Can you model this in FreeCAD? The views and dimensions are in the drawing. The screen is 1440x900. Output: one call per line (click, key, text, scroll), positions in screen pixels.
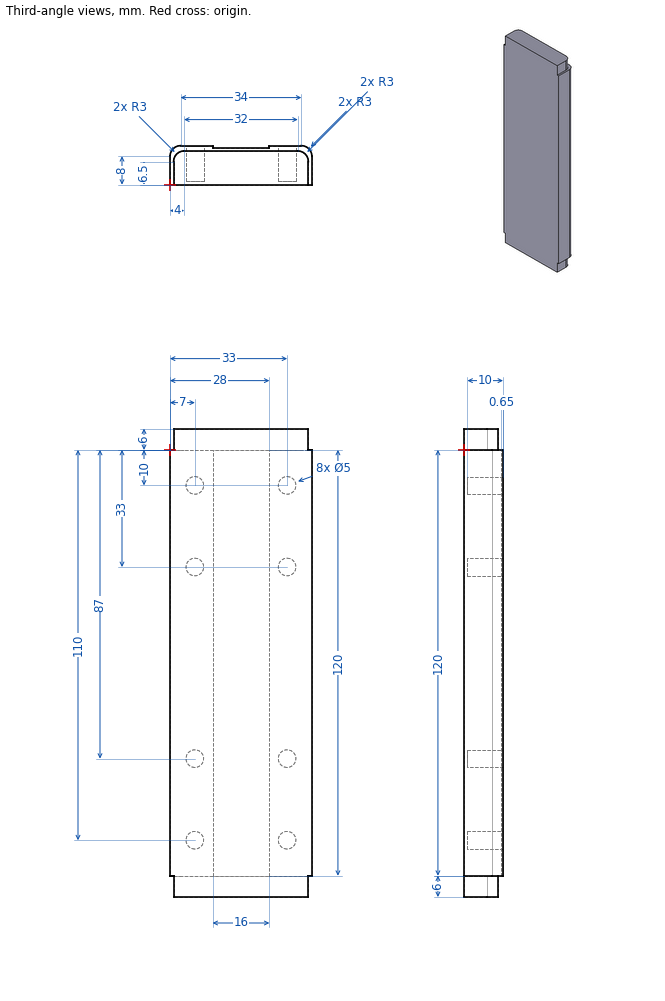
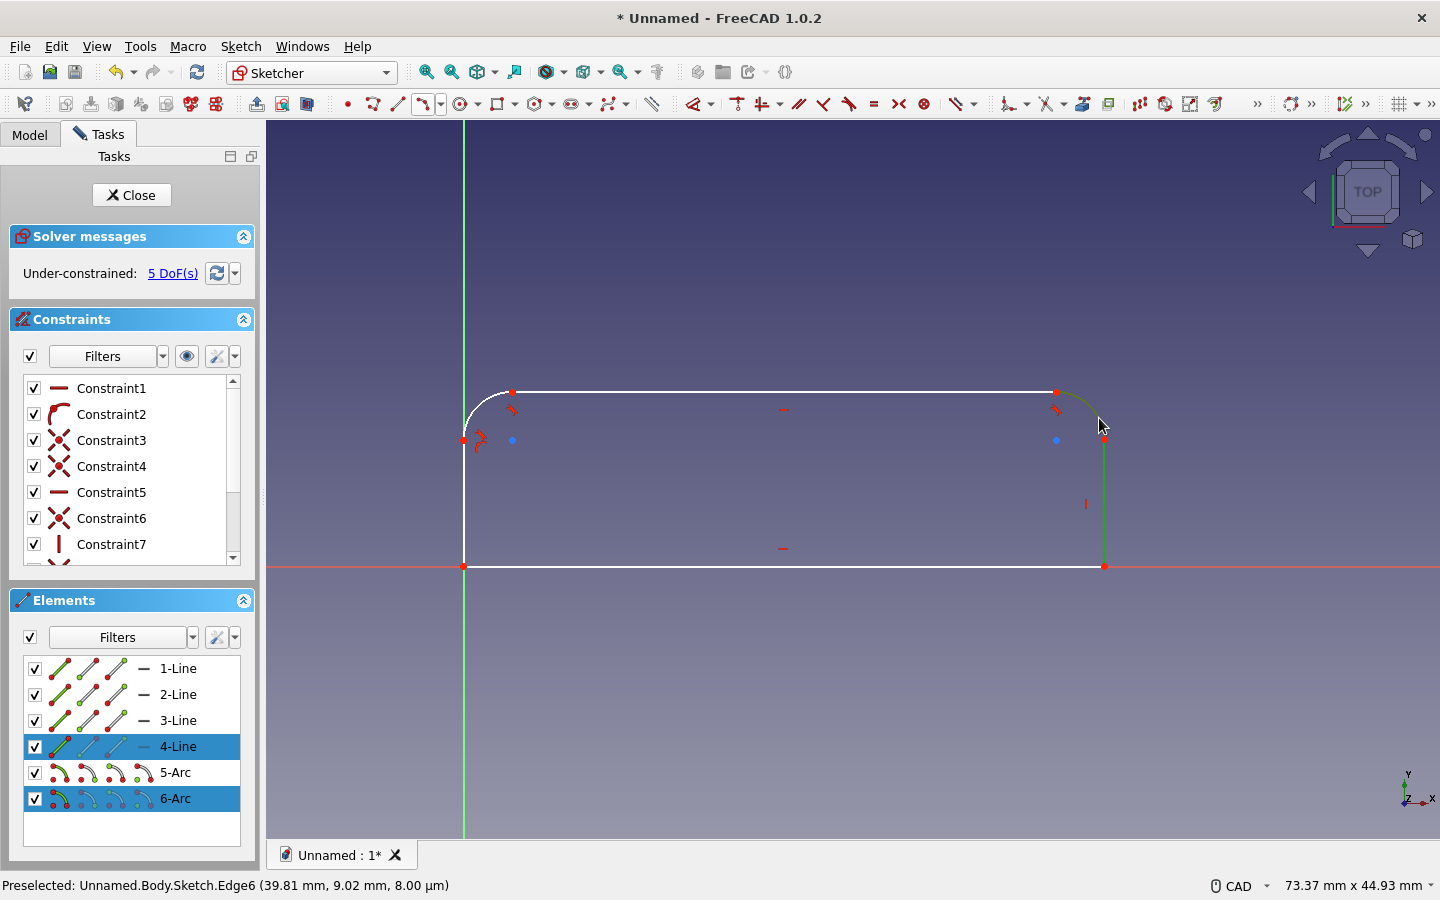
click(849, 104)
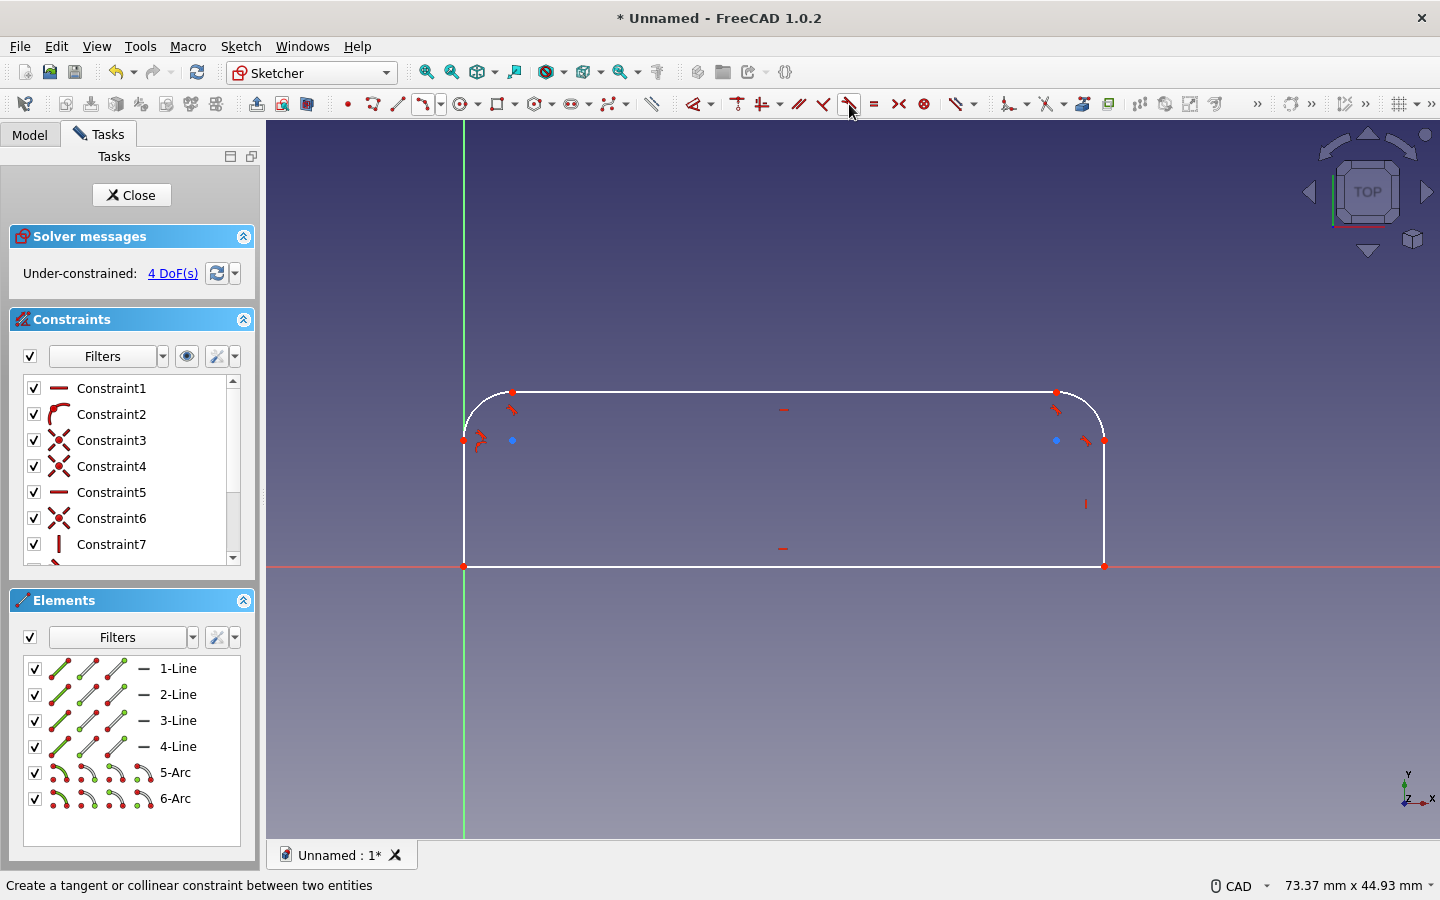
click(490, 397)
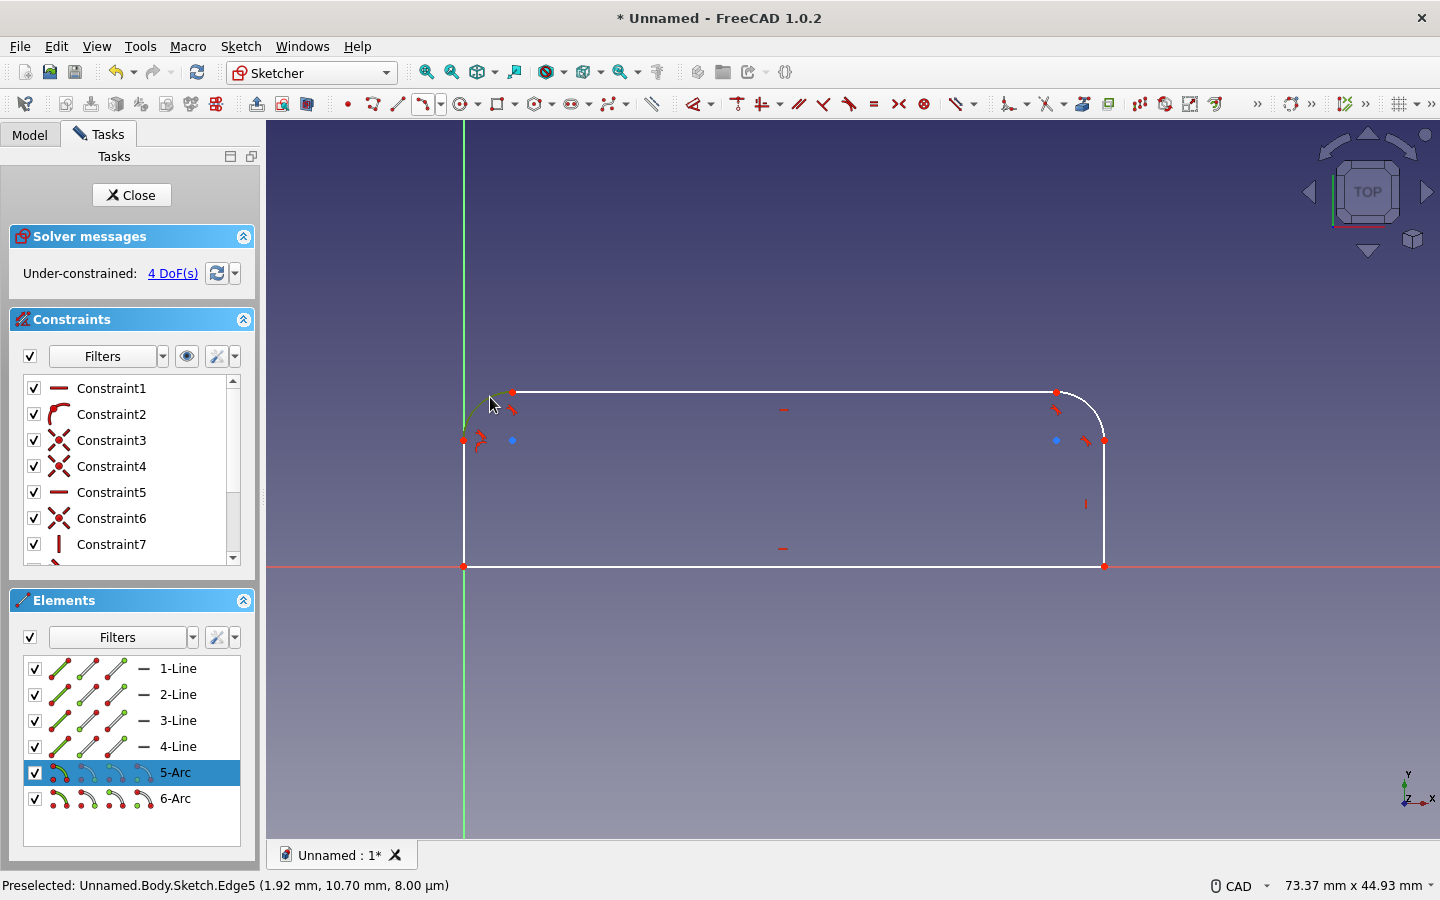
click(1099, 418)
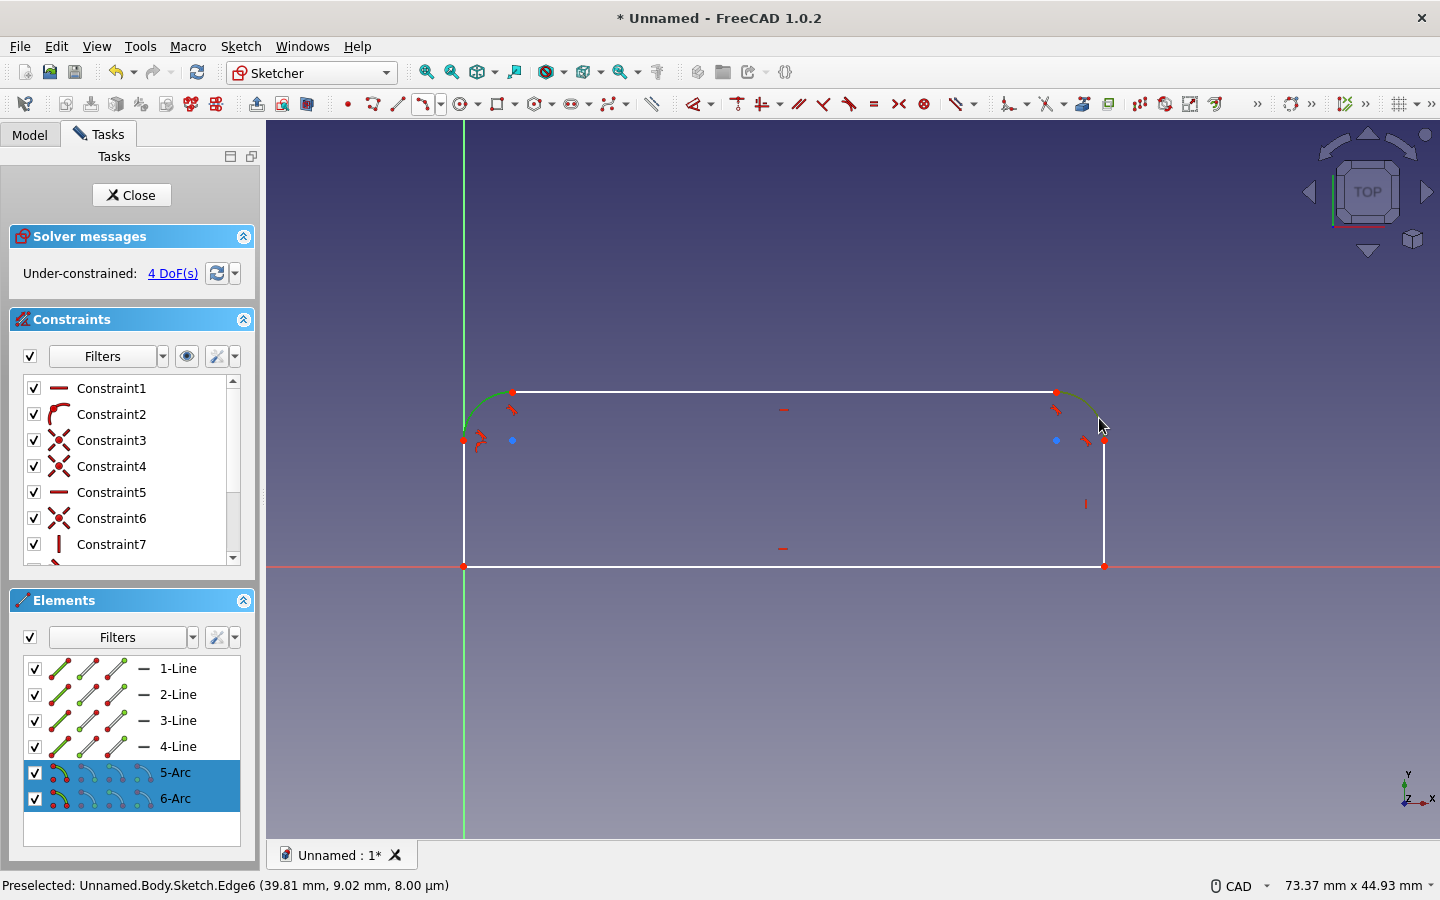
click(874, 104)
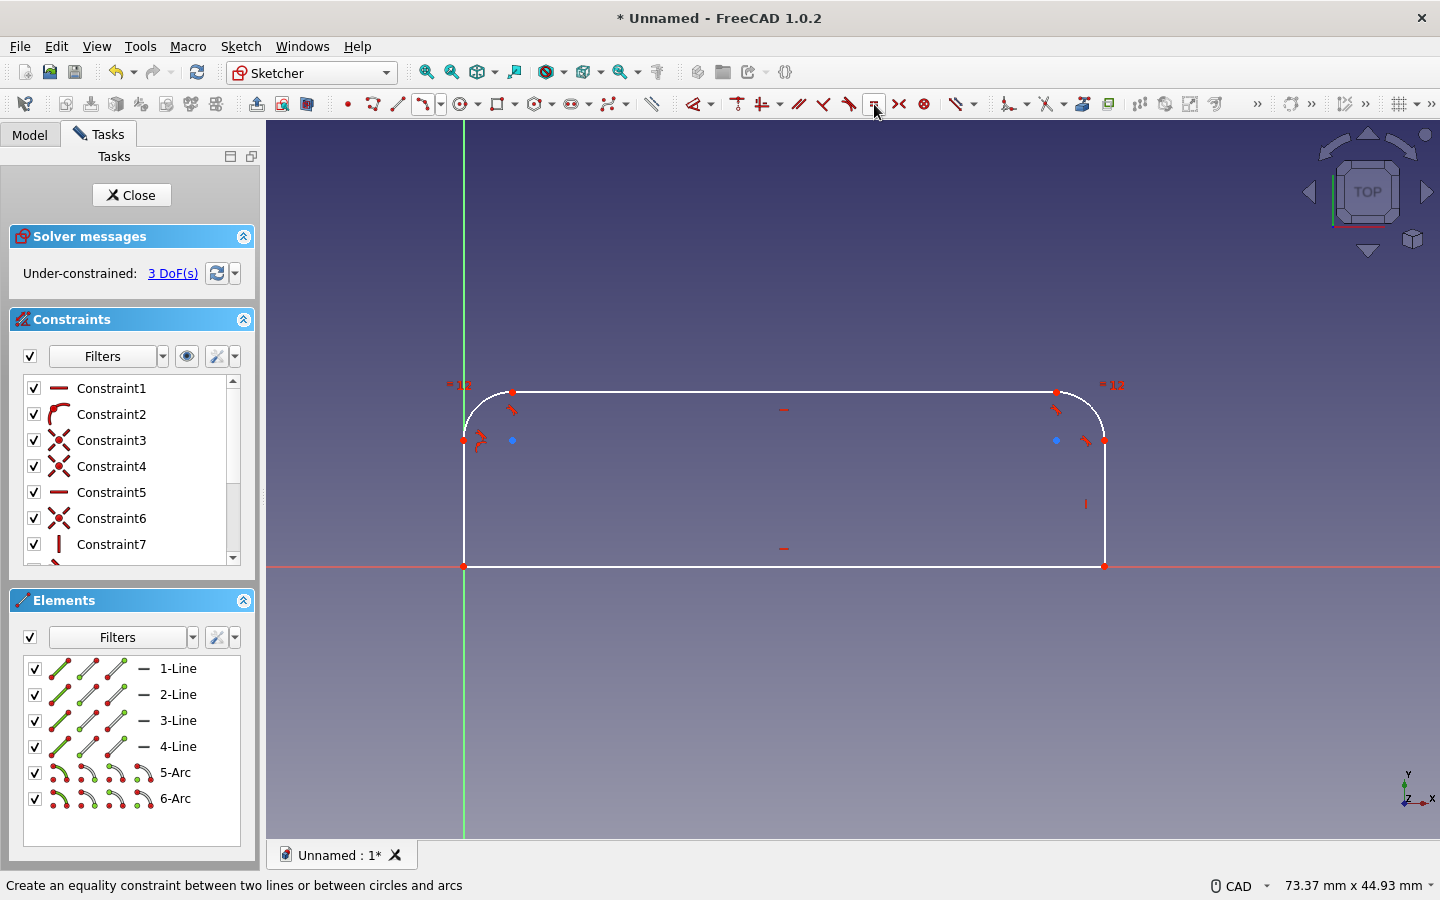
click(692, 104)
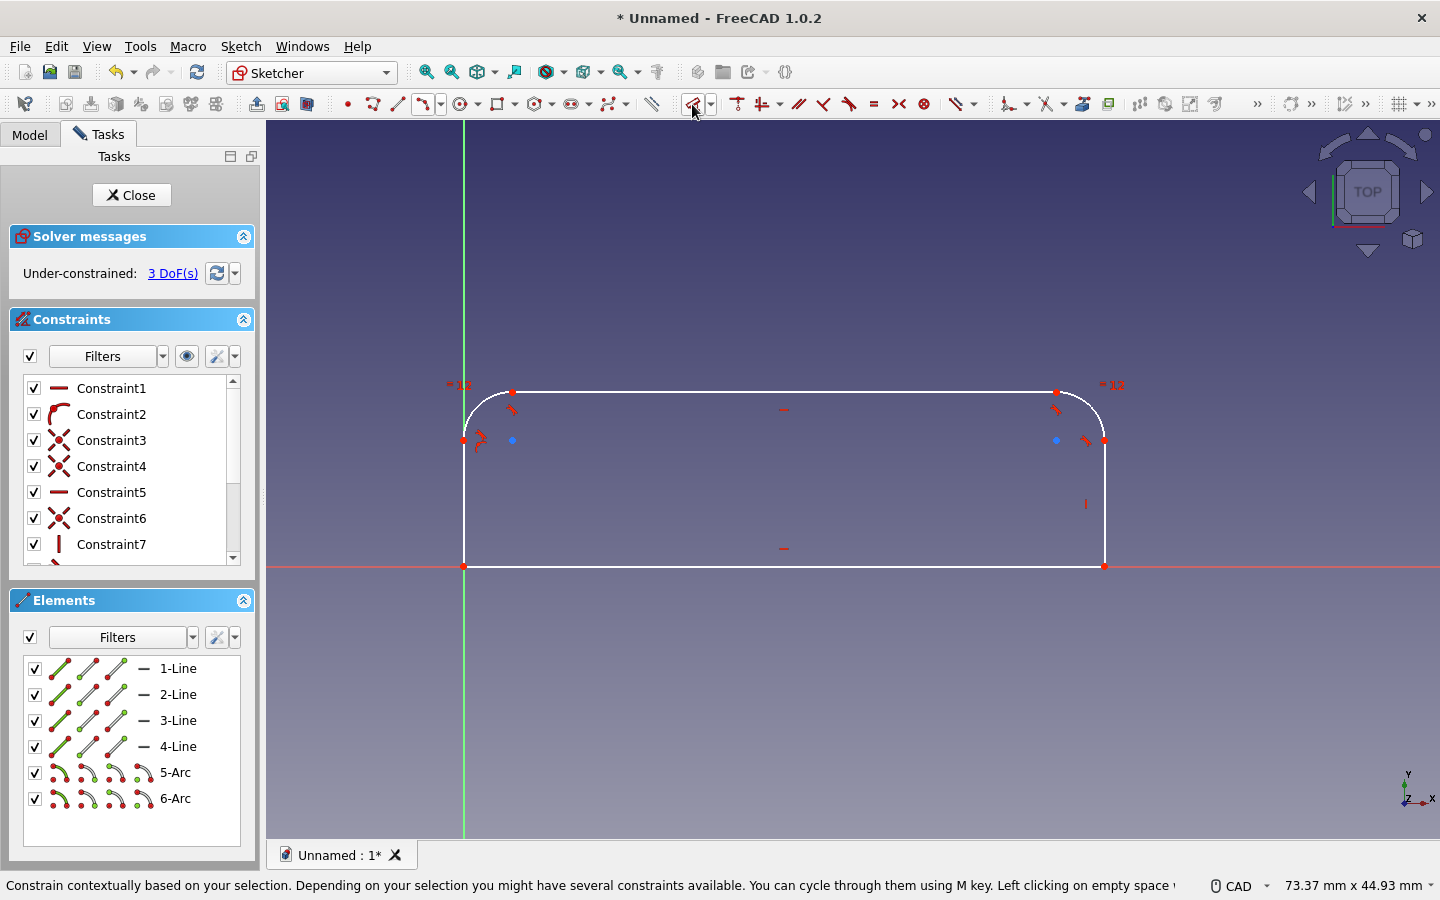
click(490, 397)
click(515, 360)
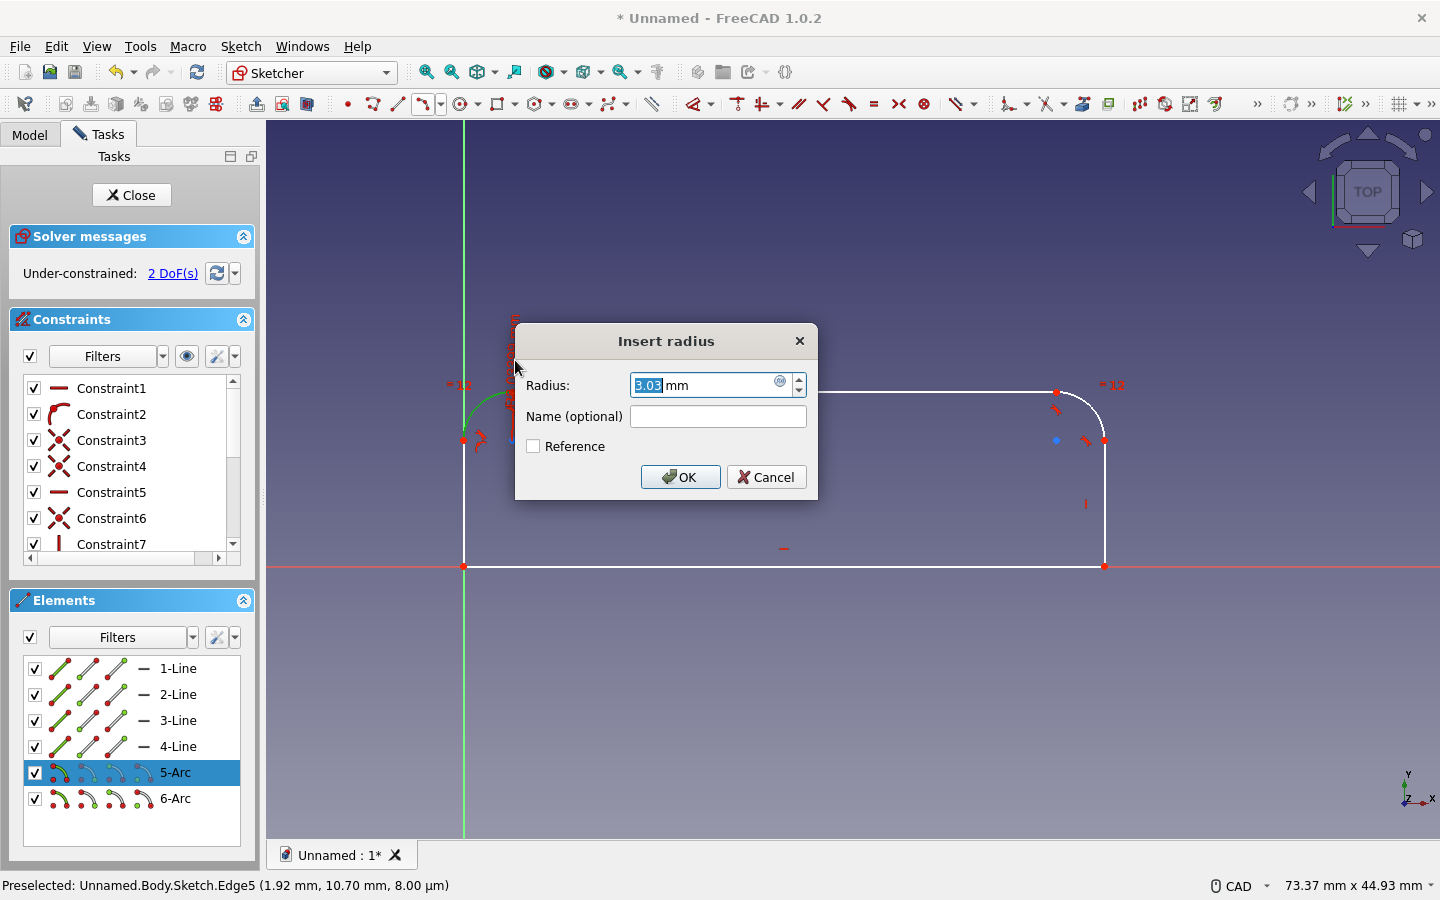
text(3)
key(Return)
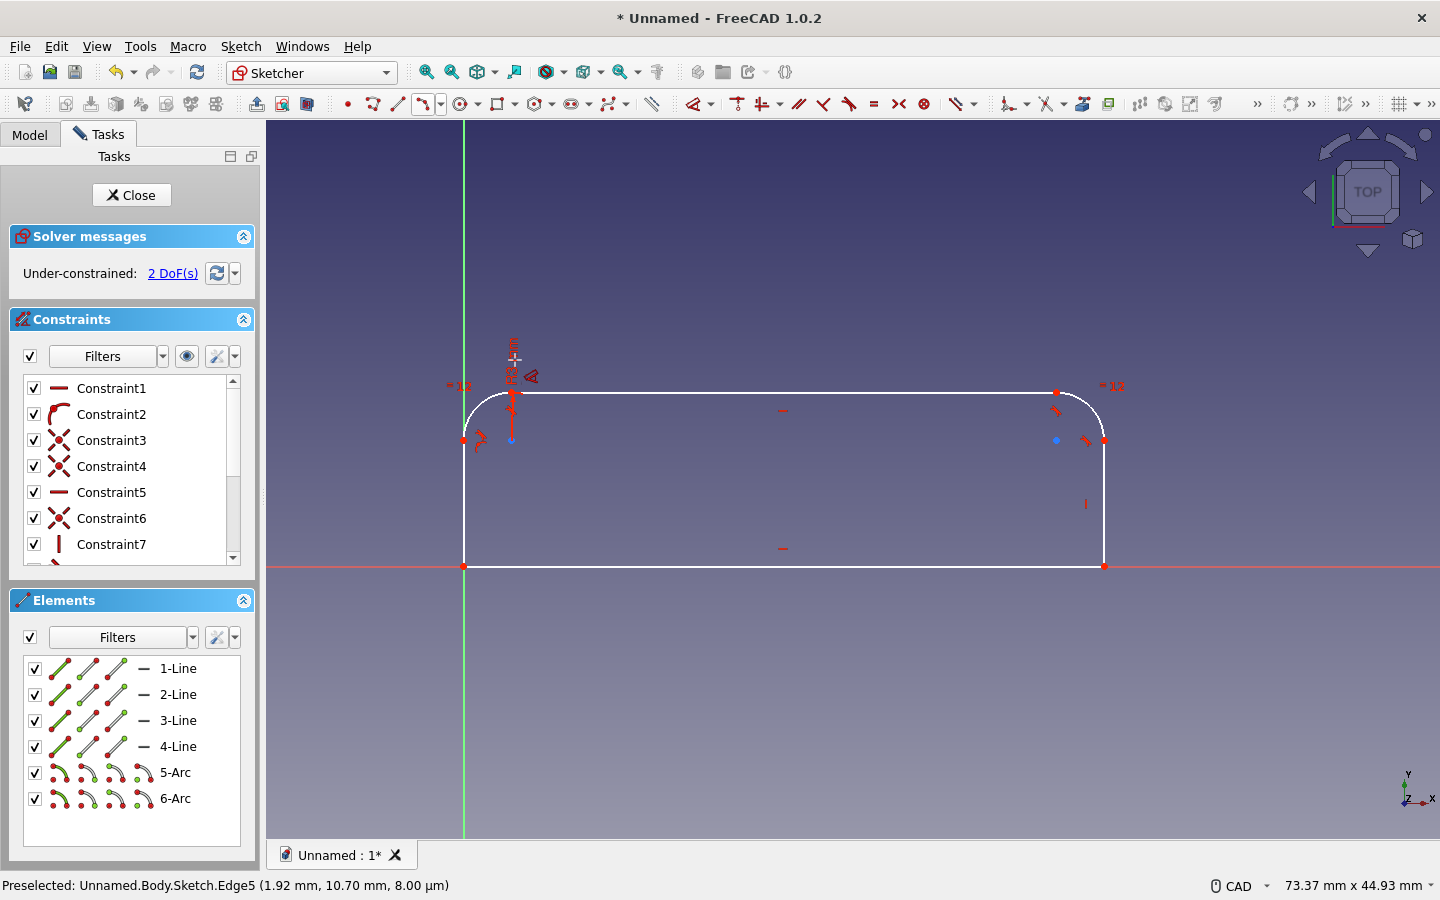
click(464, 478)
click(430, 504)